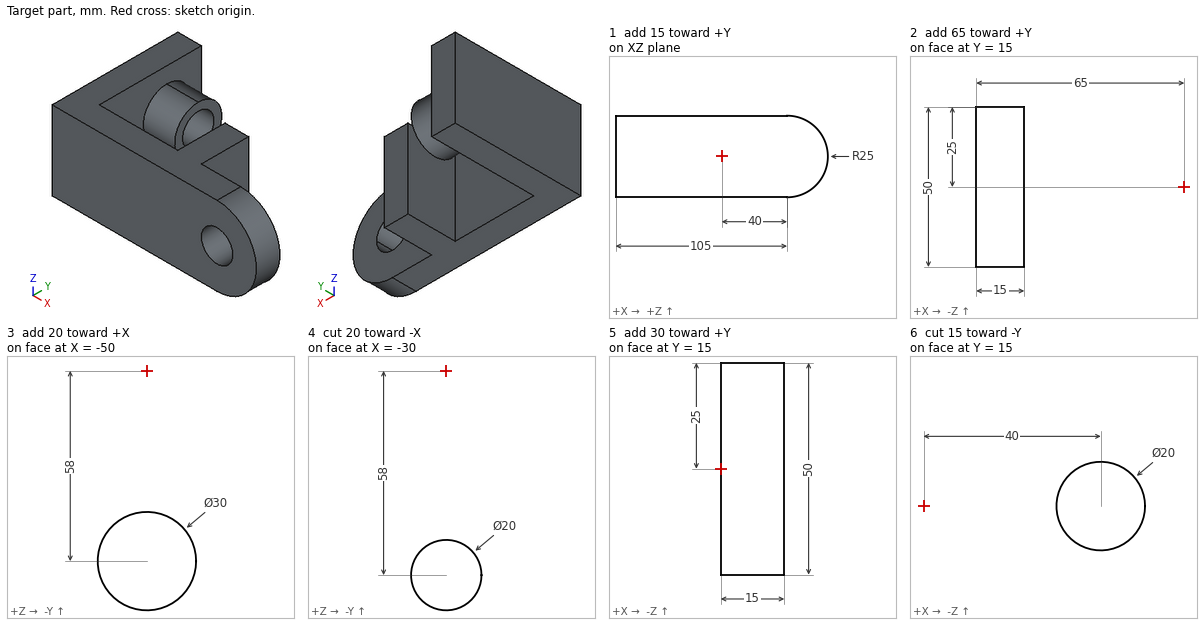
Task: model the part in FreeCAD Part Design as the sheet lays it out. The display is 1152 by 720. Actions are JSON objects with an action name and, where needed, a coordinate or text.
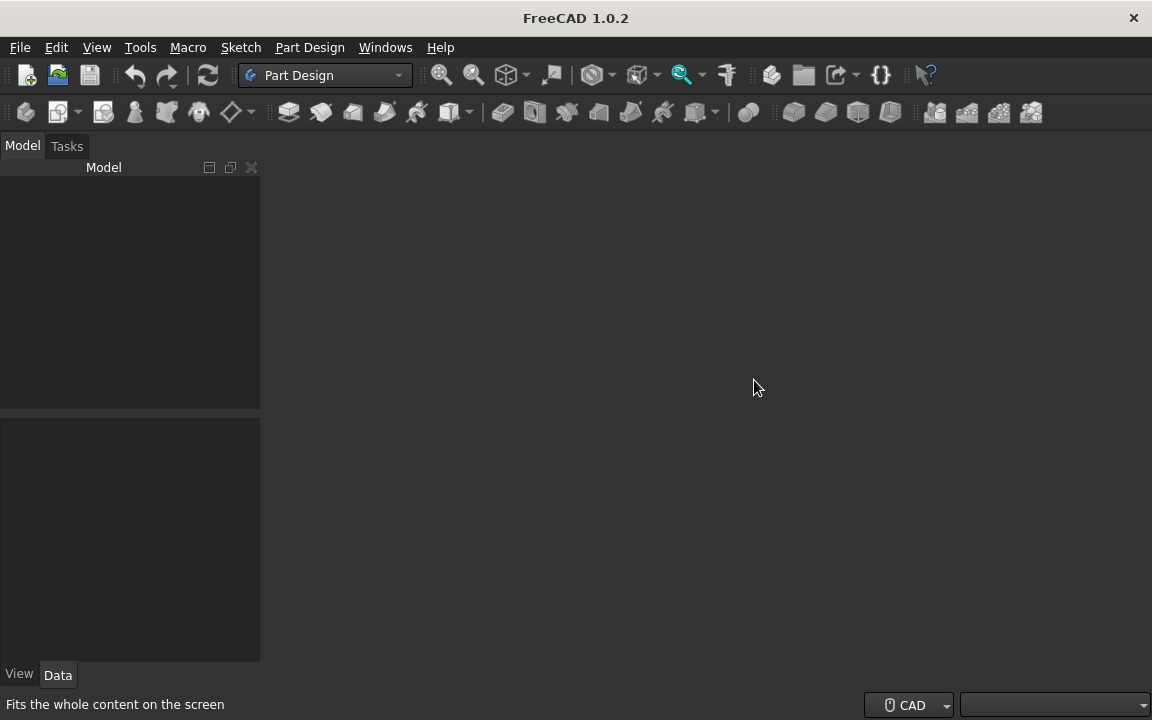
{"action": "left_click", "coordinate": [26, 76]}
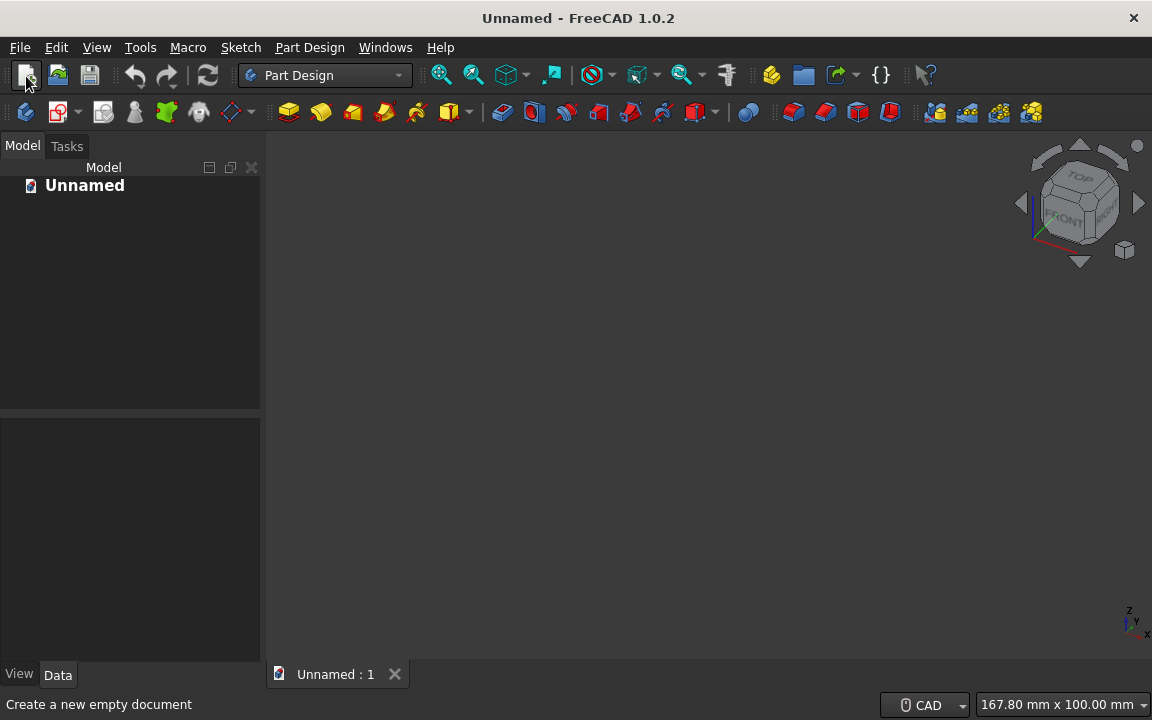
{"action": "left_click", "coordinate": [58, 112]}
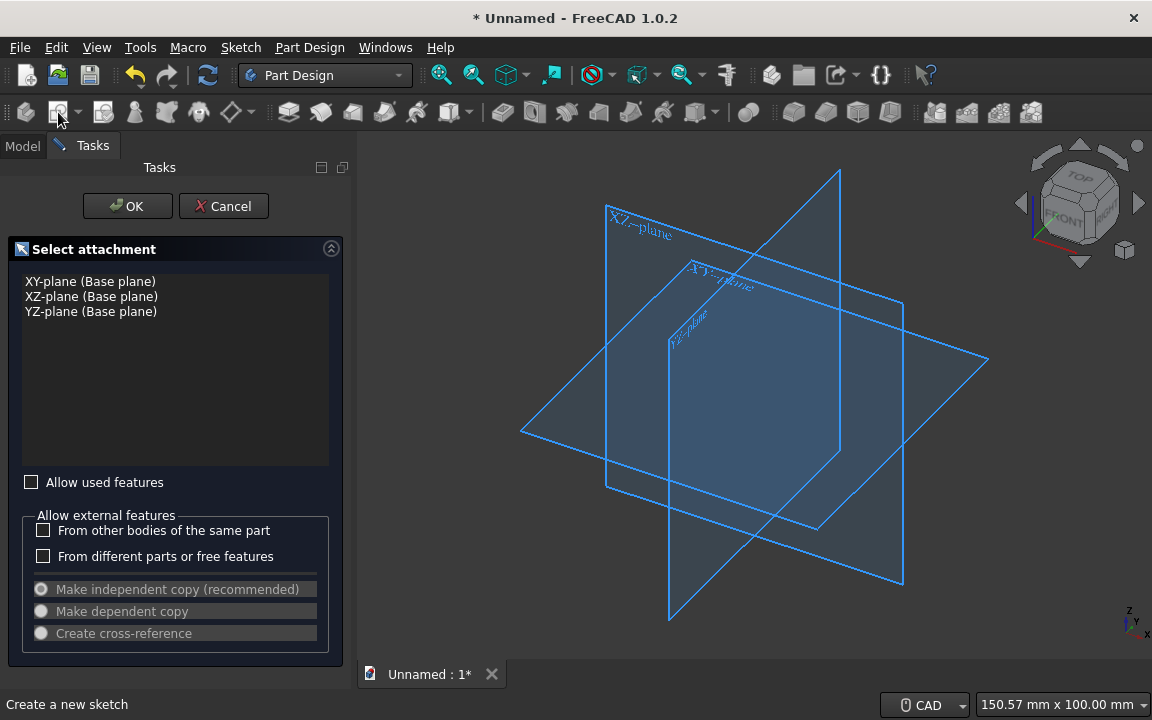
{"action": "left_click", "coordinate": [82, 296]}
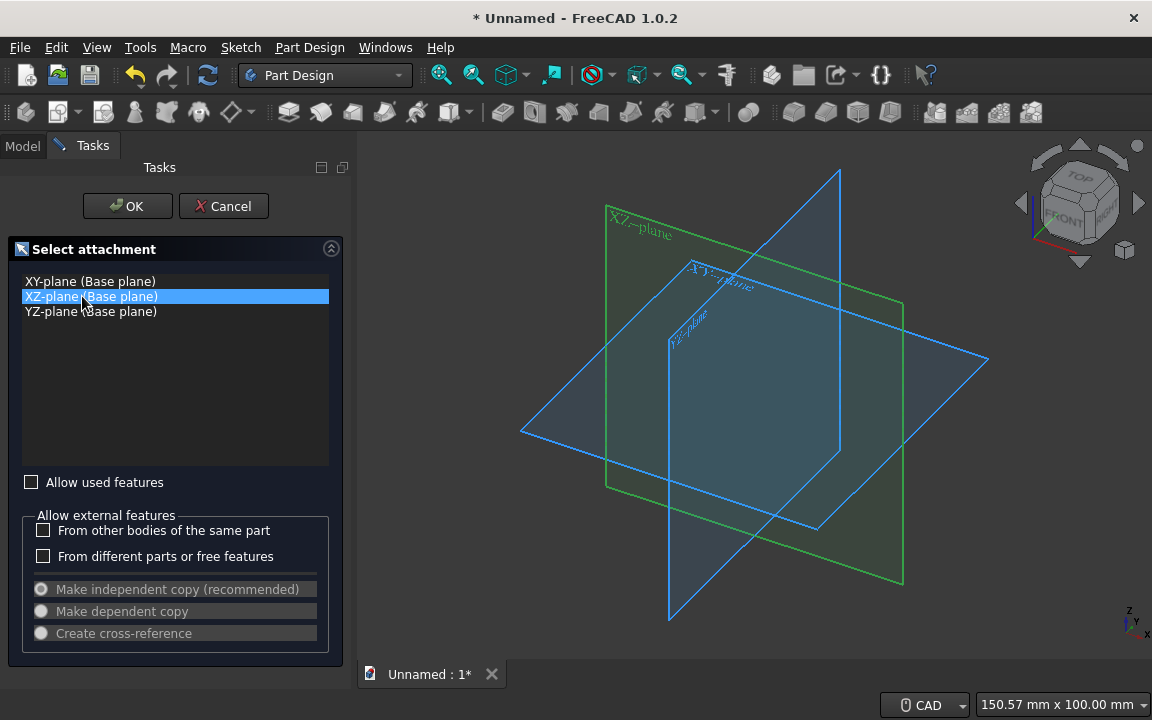
{"action": "left_click", "coordinate": [128, 206]}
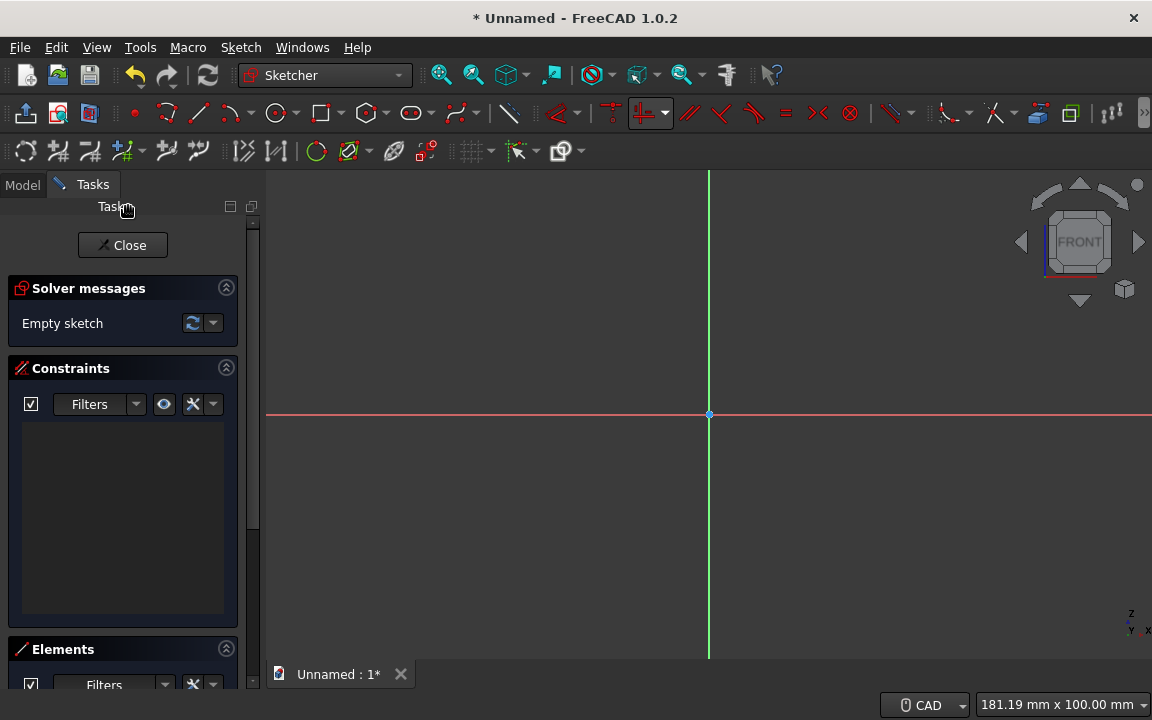
{"action": "scroll", "coordinate": [331, 415], "scroll_direction": "down", "scroll_amount": 1}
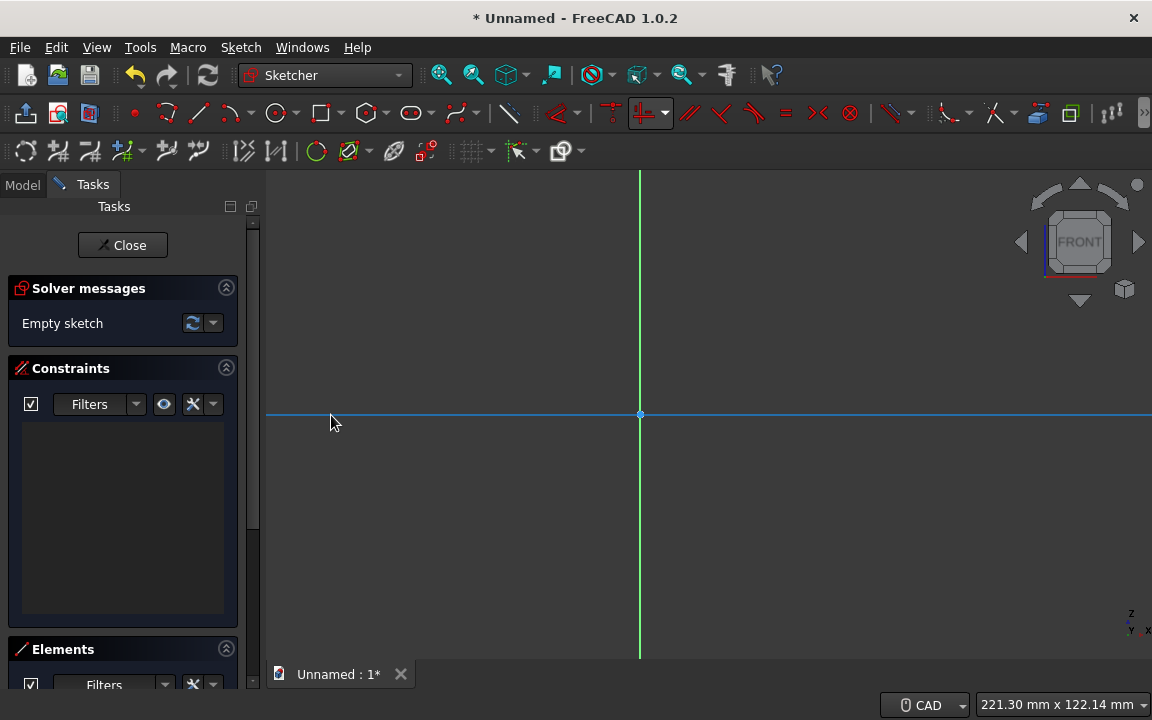
{"action": "left_click", "coordinate": [168, 114]}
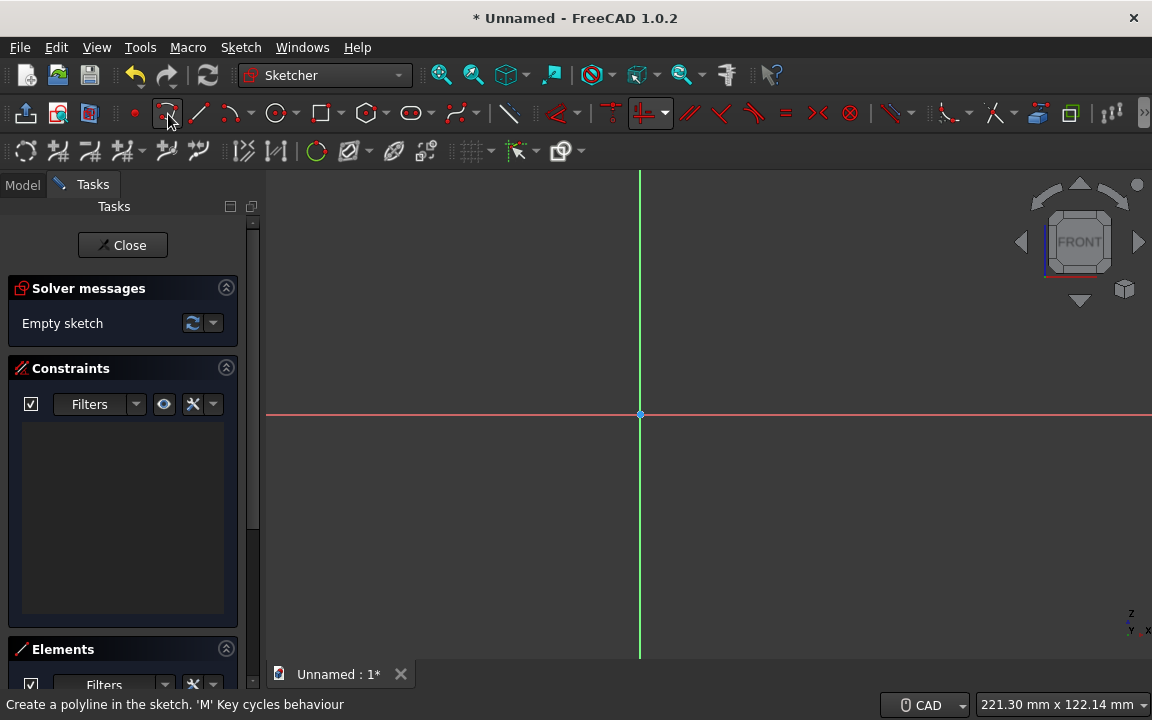
{"action": "left_click", "coordinate": [801, 515]}
{"action": "left_click", "coordinate": [380, 515]}
{"action": "left_click", "coordinate": [380, 315]}
{"action": "left_click", "coordinate": [801, 315]}
{"action": "right_click", "coordinate": [801, 315]}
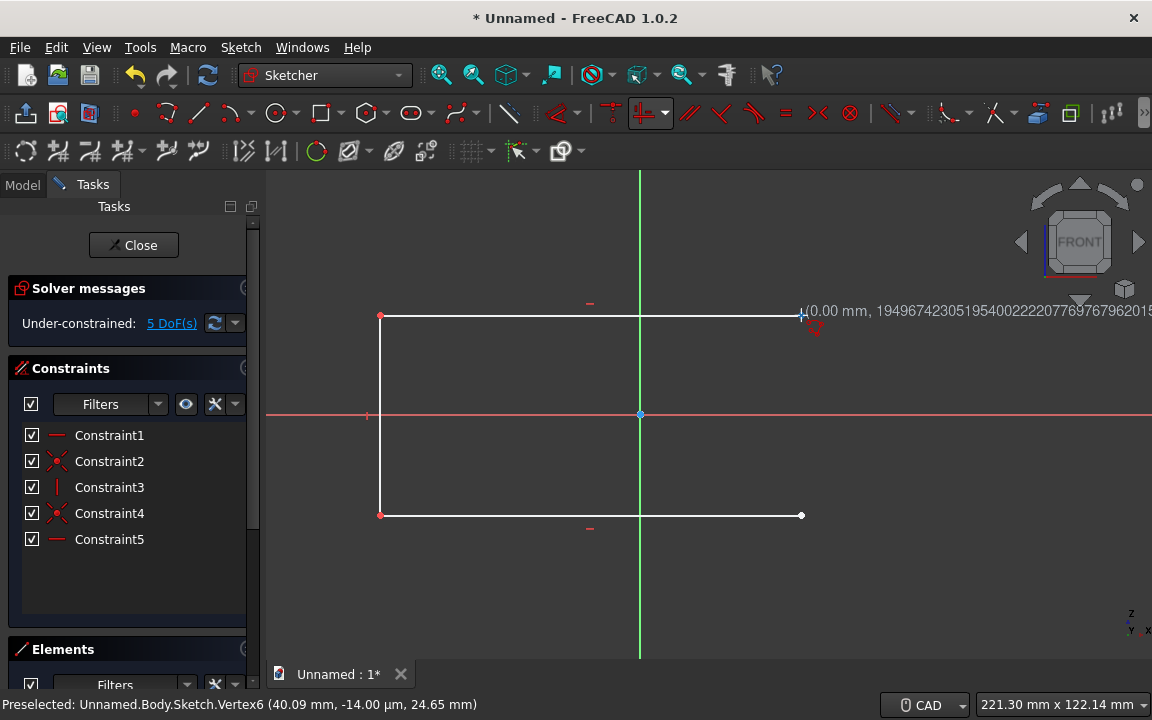
{"action": "left_click", "coordinate": [254, 114]}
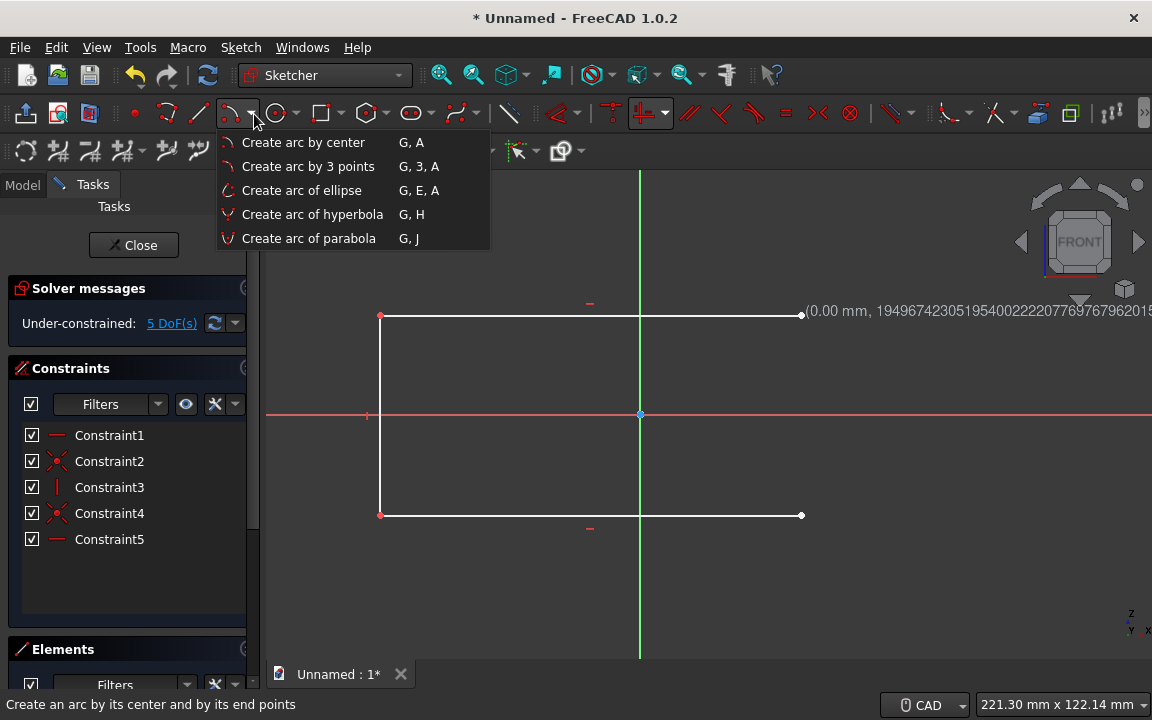
{"action": "left_click", "coordinate": [354, 166]}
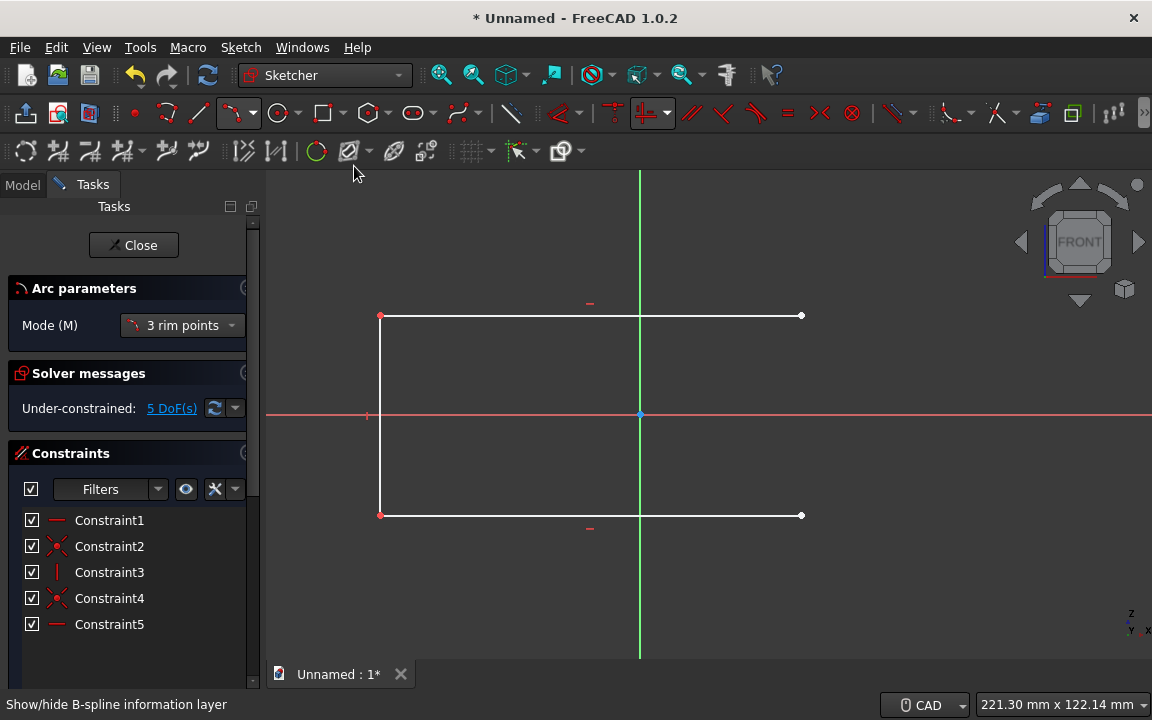
{"action": "left_click", "coordinate": [801, 316]}
{"action": "left_click", "coordinate": [801, 516]}
{"action": "left_click", "coordinate": [896, 446]}
{"action": "key", "text": "Escape"}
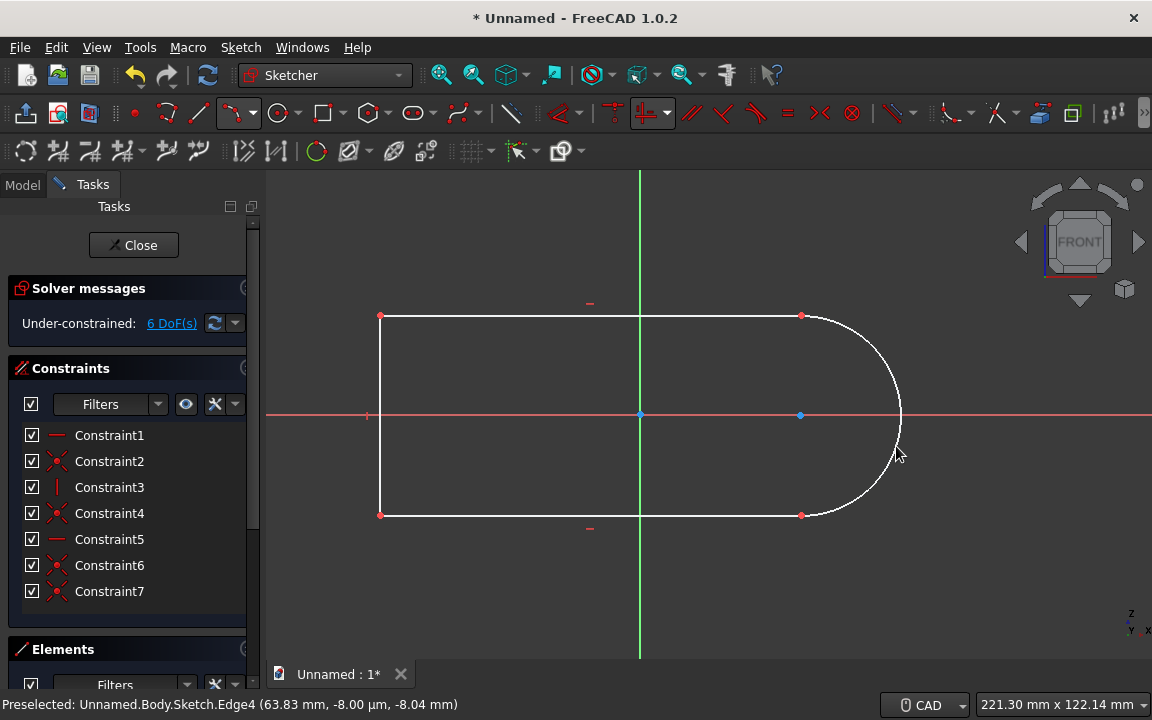
{"action": "left_click", "coordinate": [675, 516]}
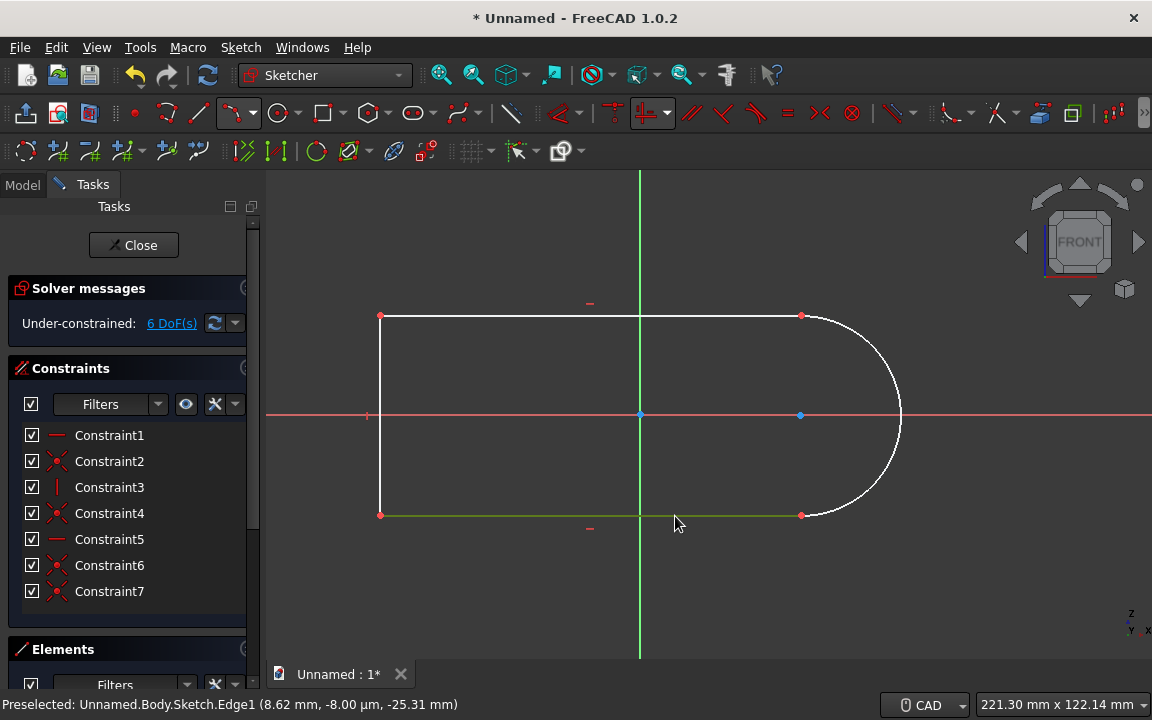
{"action": "left_click", "coordinate": [882, 475]}